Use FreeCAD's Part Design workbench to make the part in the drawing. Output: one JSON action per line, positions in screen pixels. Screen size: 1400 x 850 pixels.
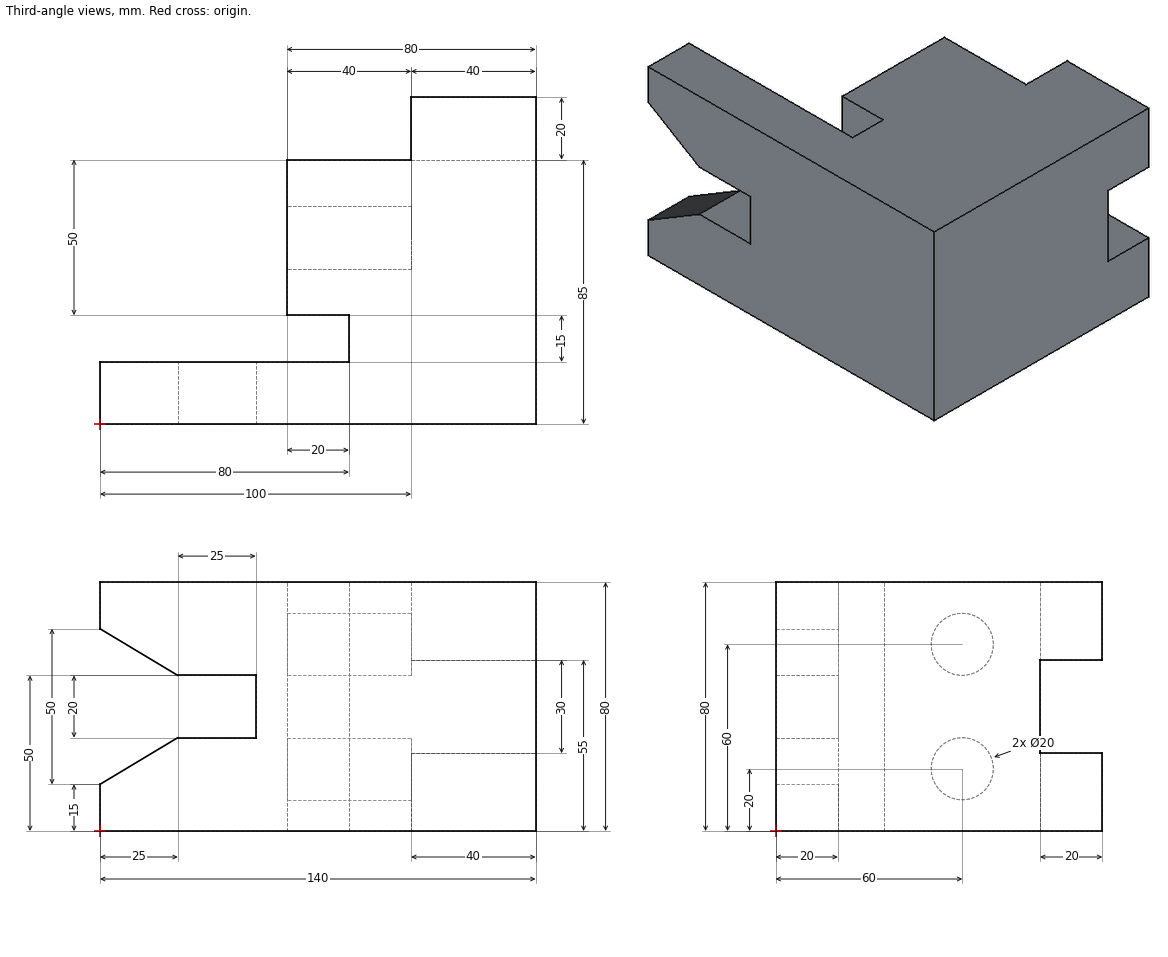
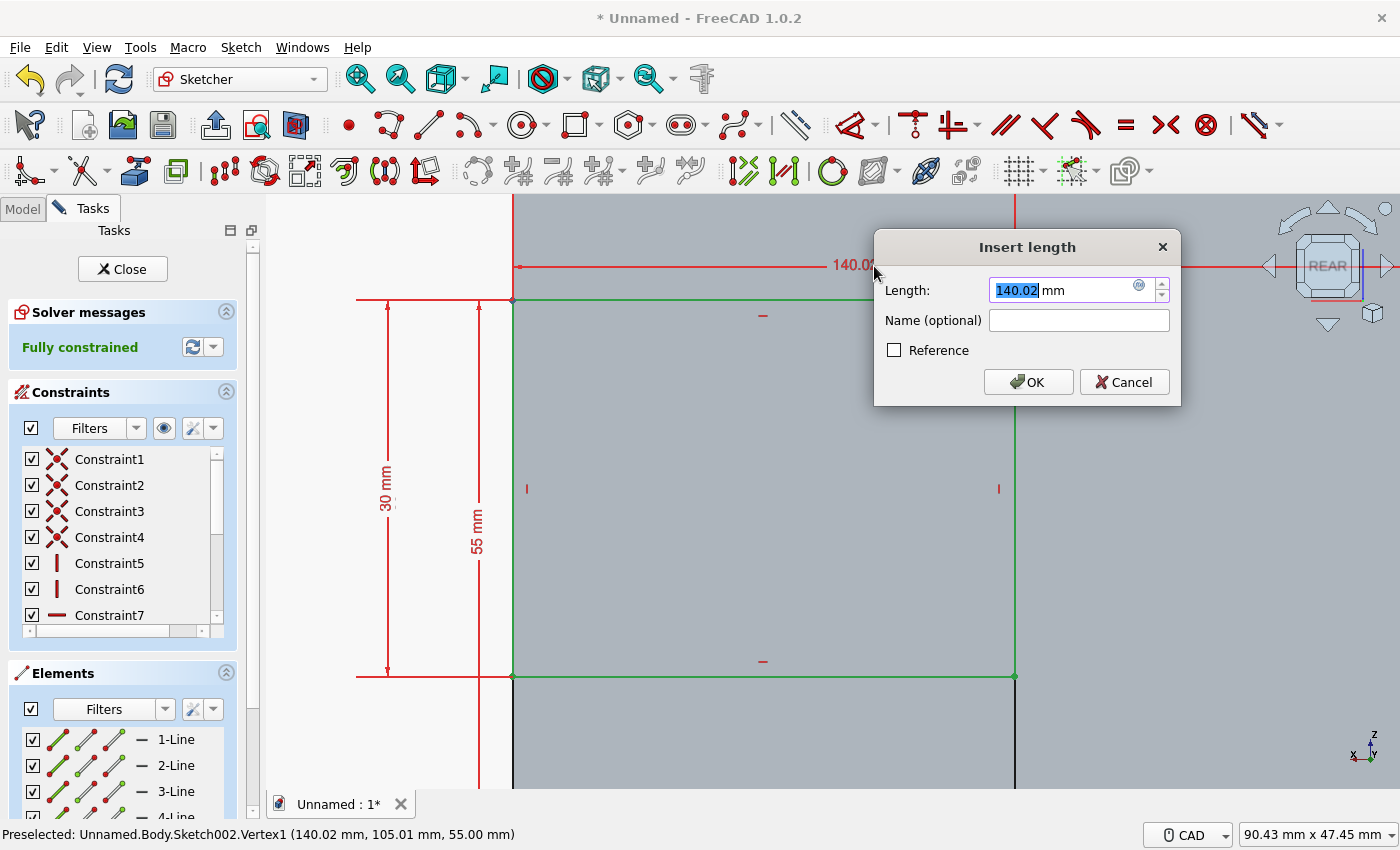
{"action": "type", "text": "140"}
{"action": "key", "text": "Return"}
{"action": "key", "text": "Escape"}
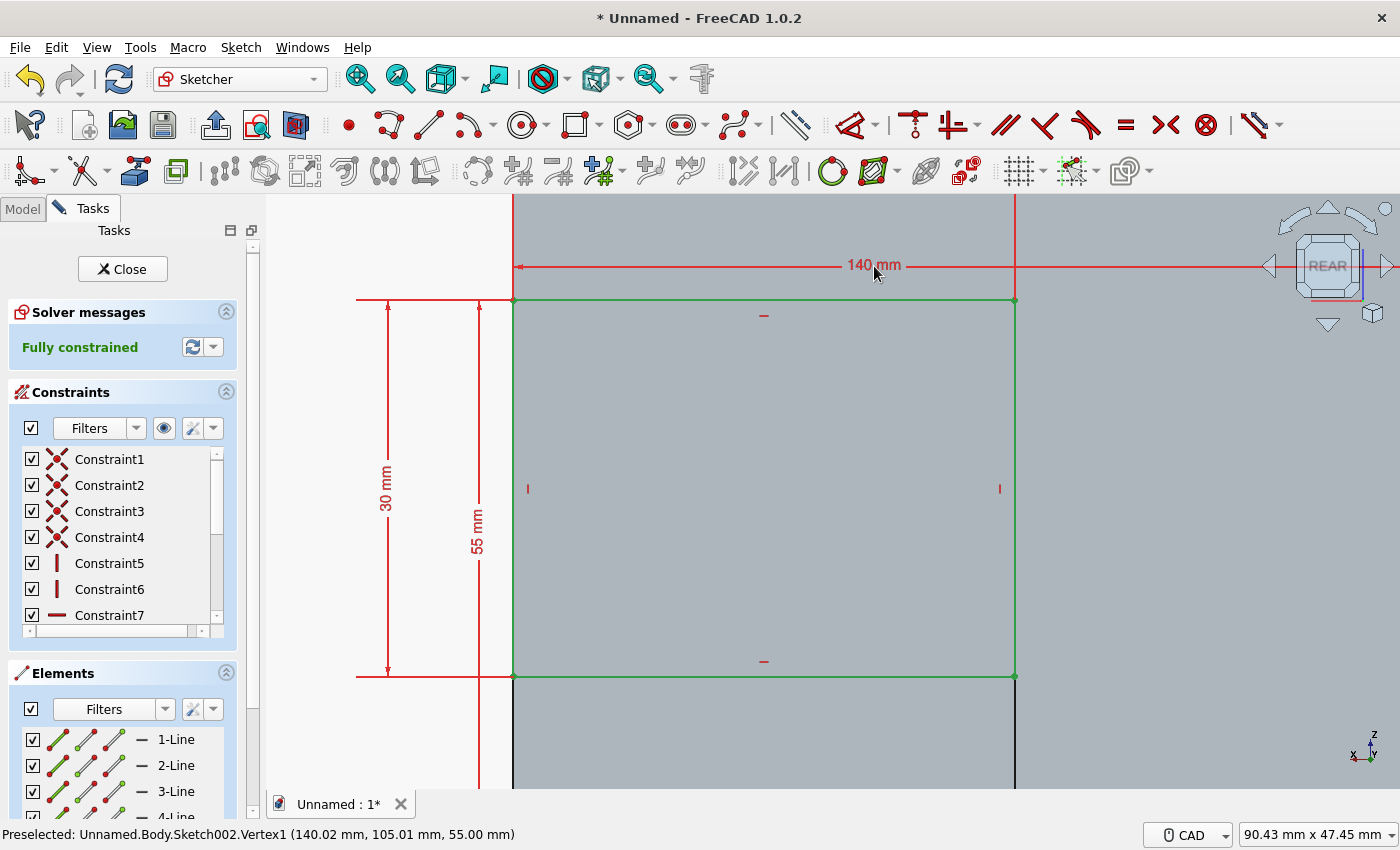
{"action": "left_click", "coordinate": [123, 269]}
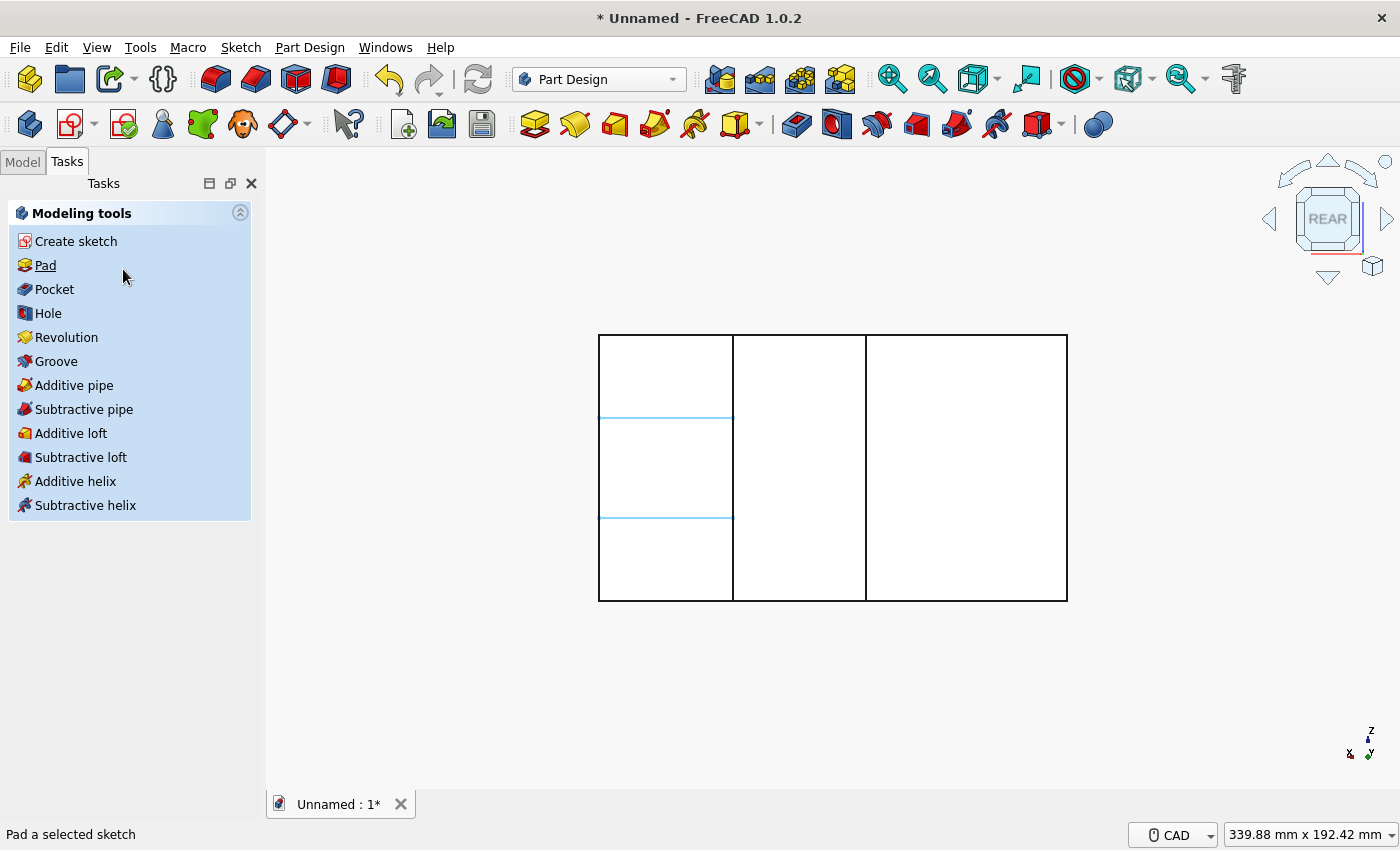
{"action": "left_click", "coordinate": [798, 124]}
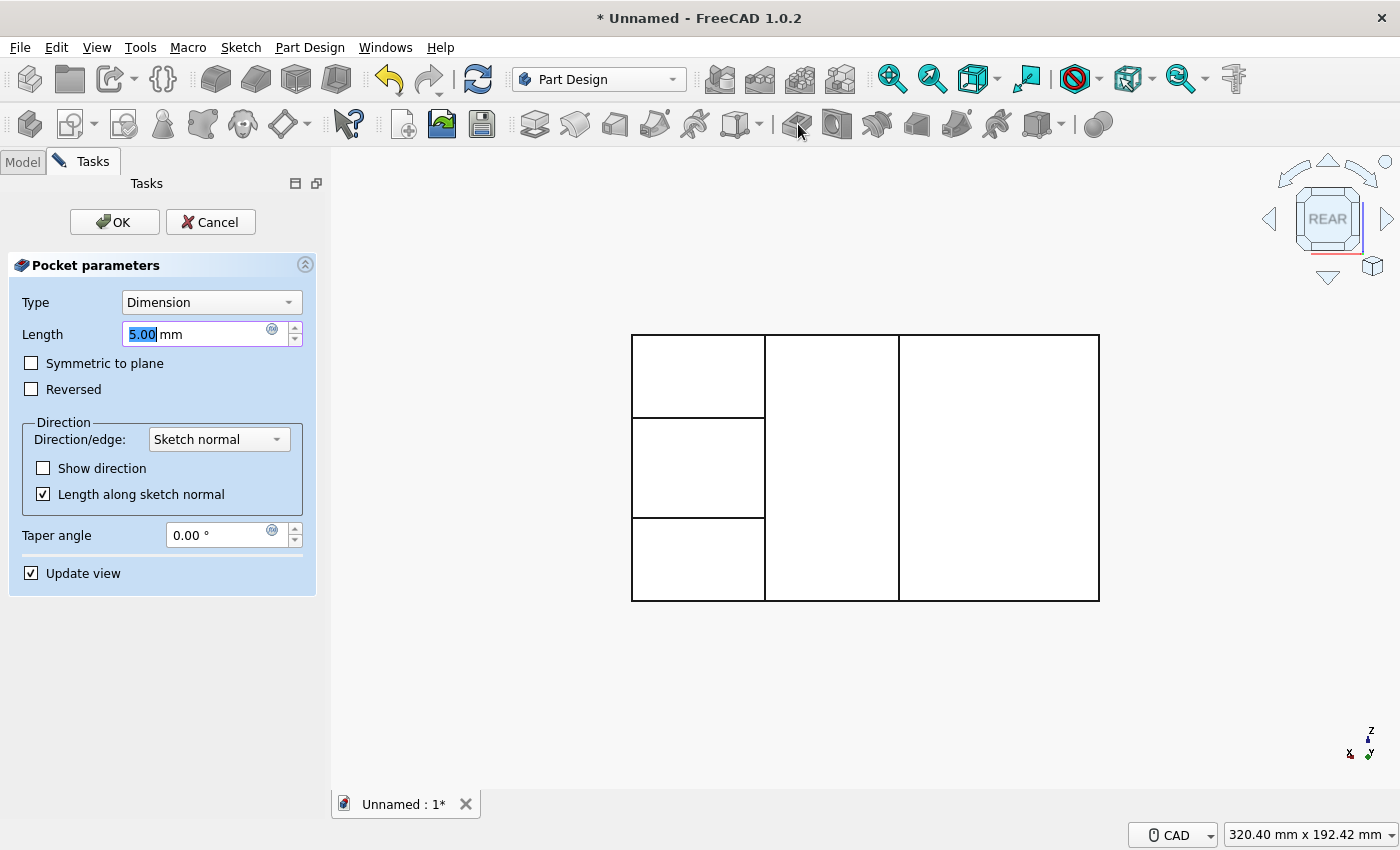
{"action": "type", "text": "20"}
{"action": "key", "text": "Tab"}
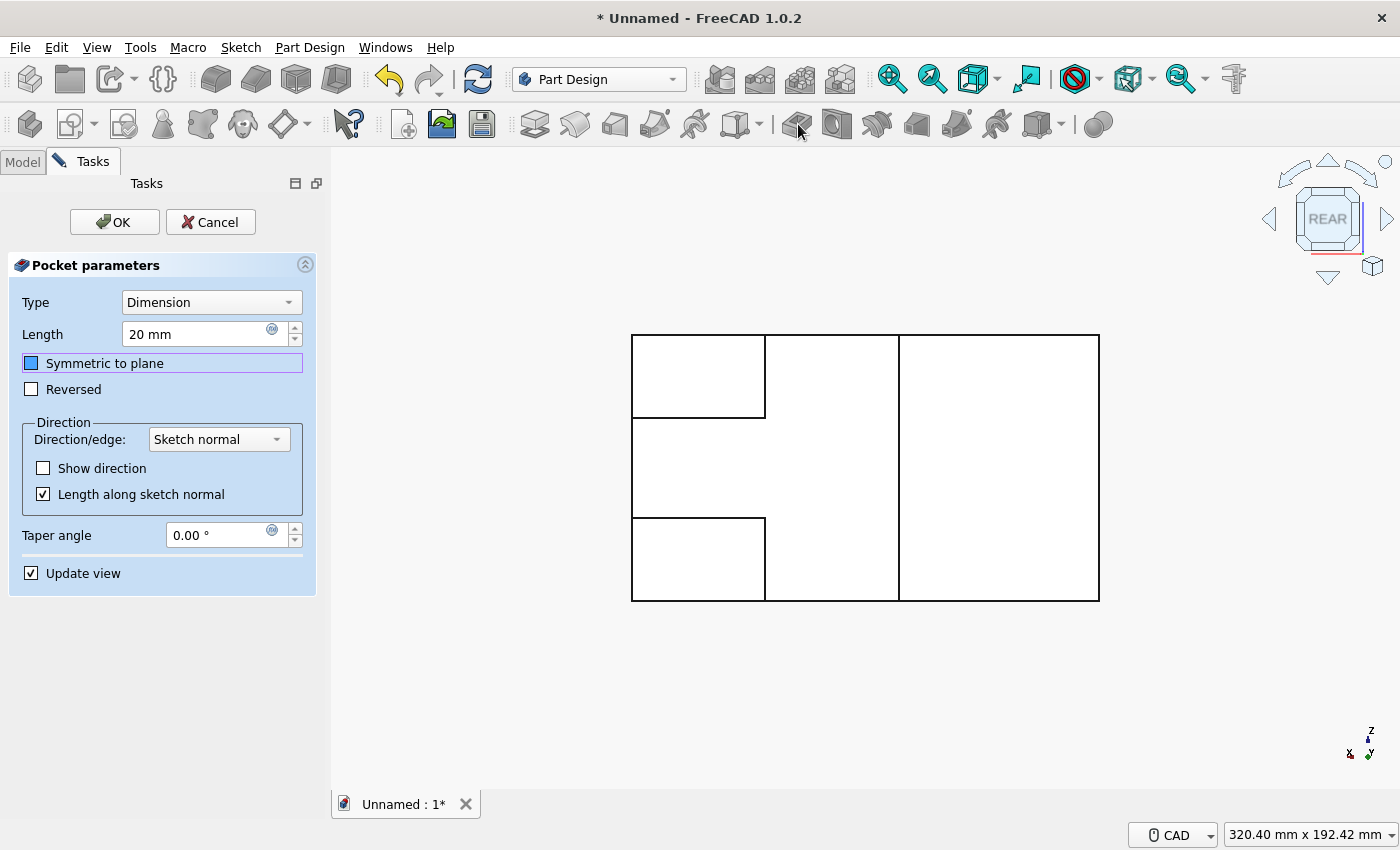
{"action": "left_click", "coordinate": [115, 222]}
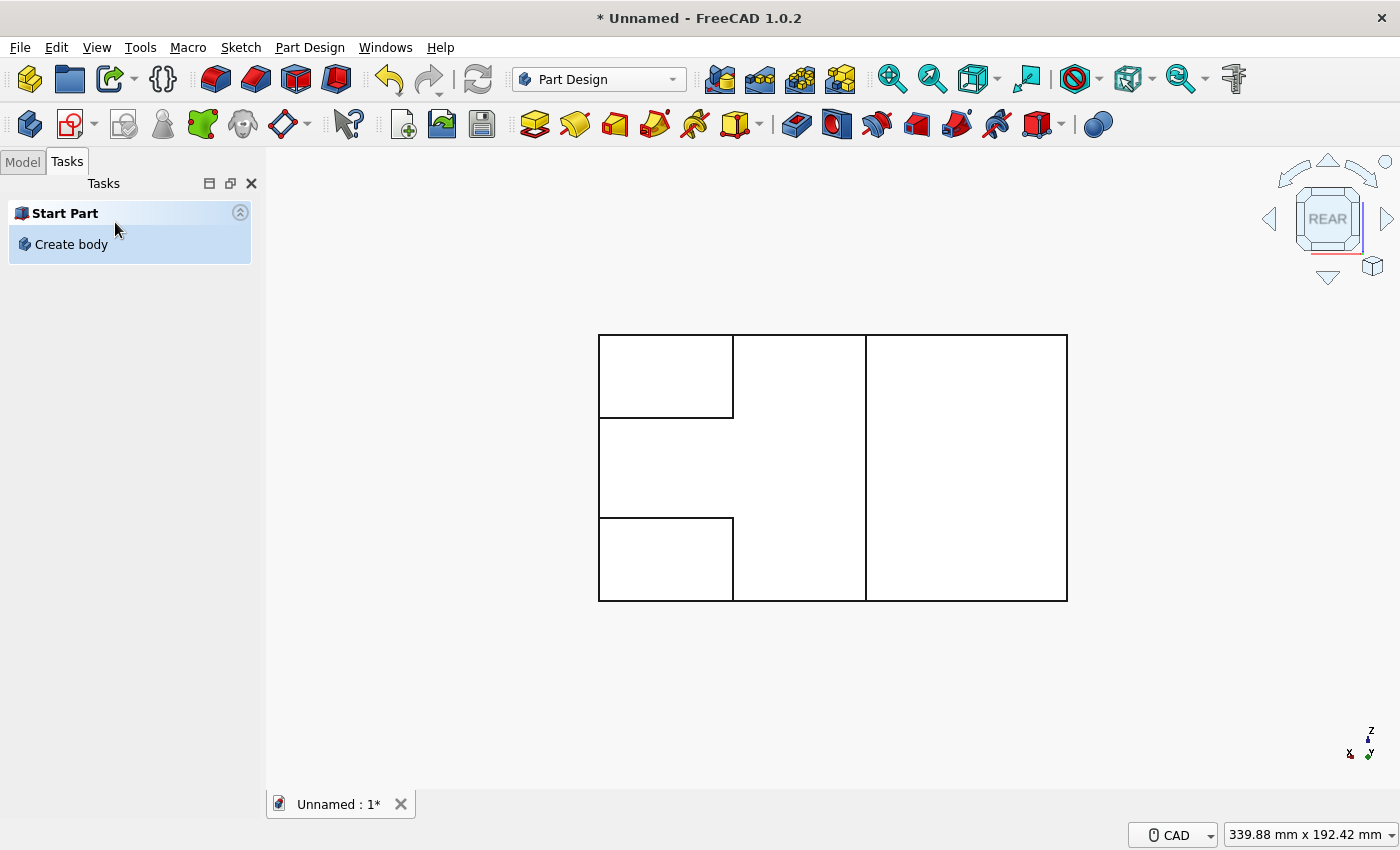
{"action": "key", "text": "v f"}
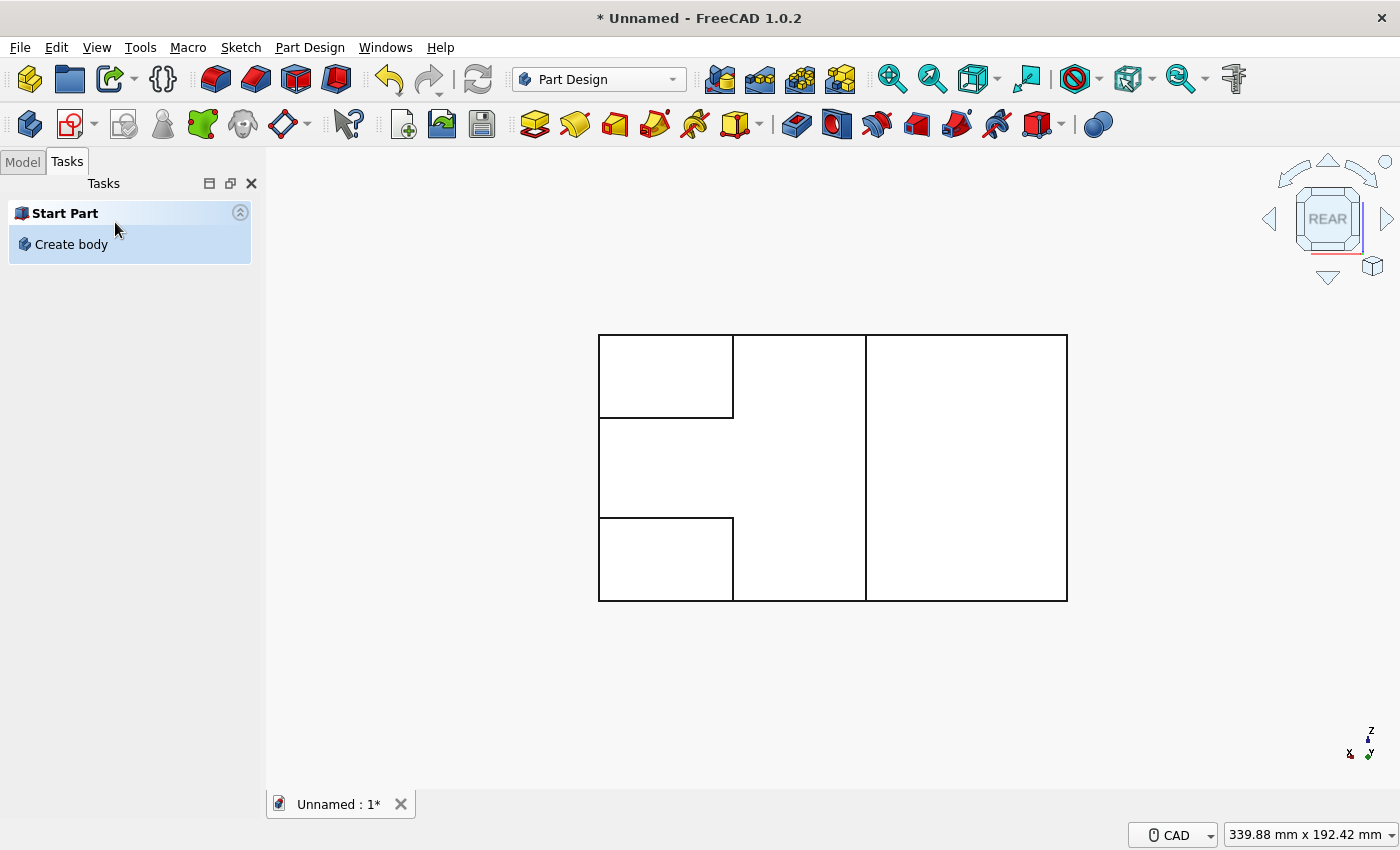
{"action": "left_click", "coordinate": [933, 467]}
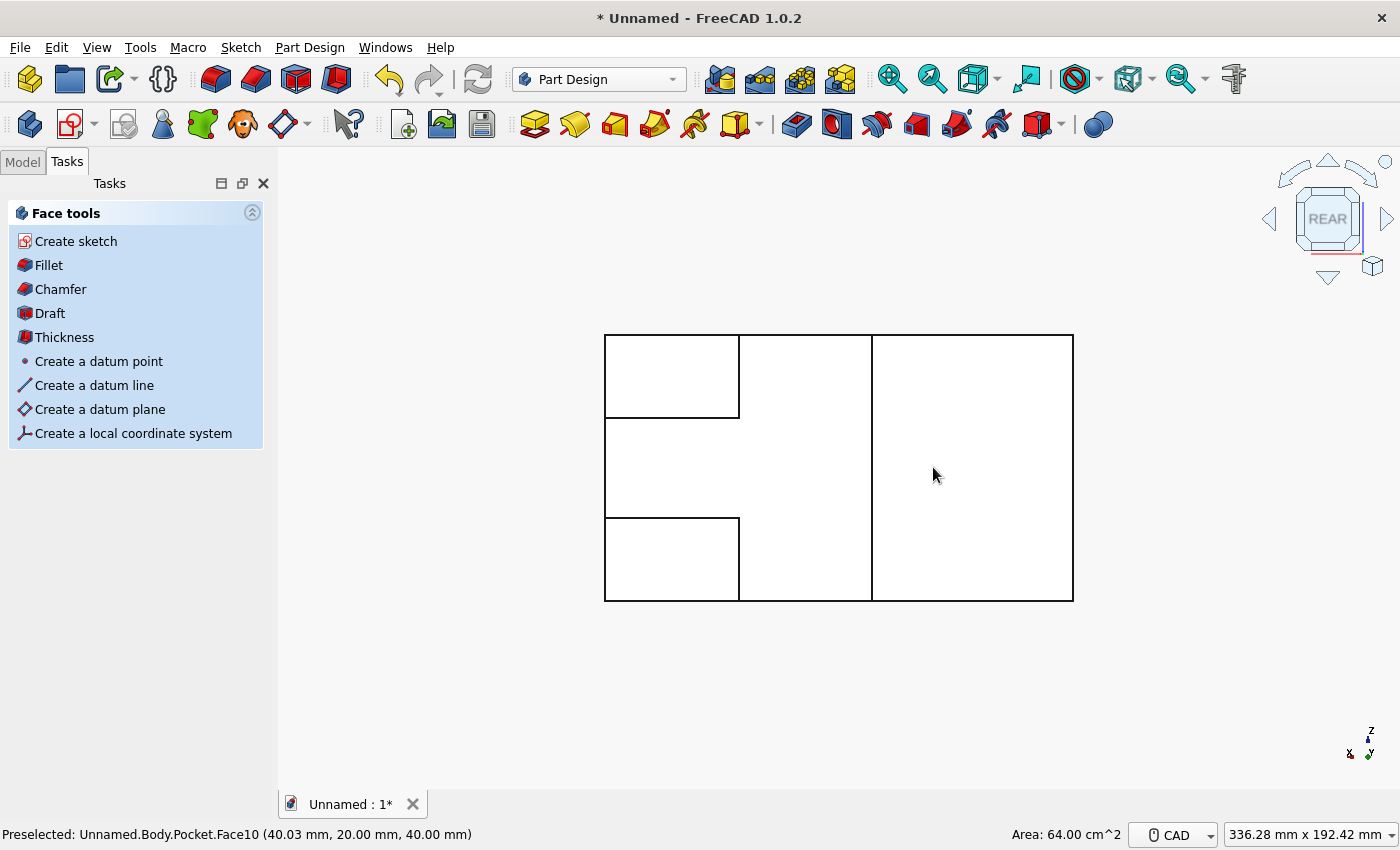
{"action": "left_click", "coordinate": [70, 124]}